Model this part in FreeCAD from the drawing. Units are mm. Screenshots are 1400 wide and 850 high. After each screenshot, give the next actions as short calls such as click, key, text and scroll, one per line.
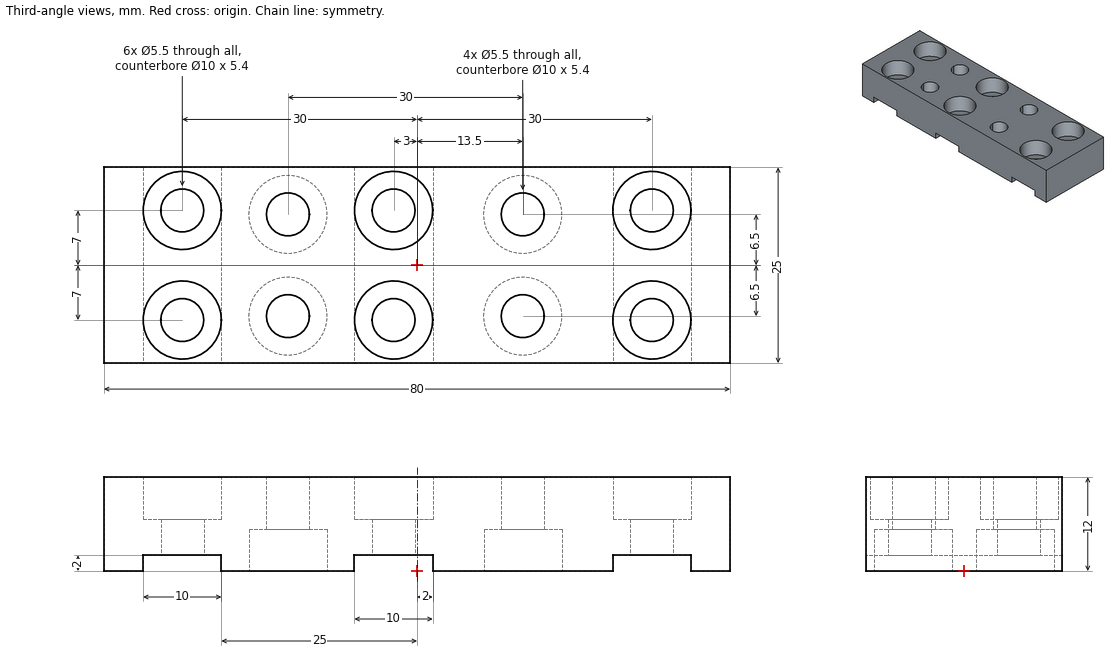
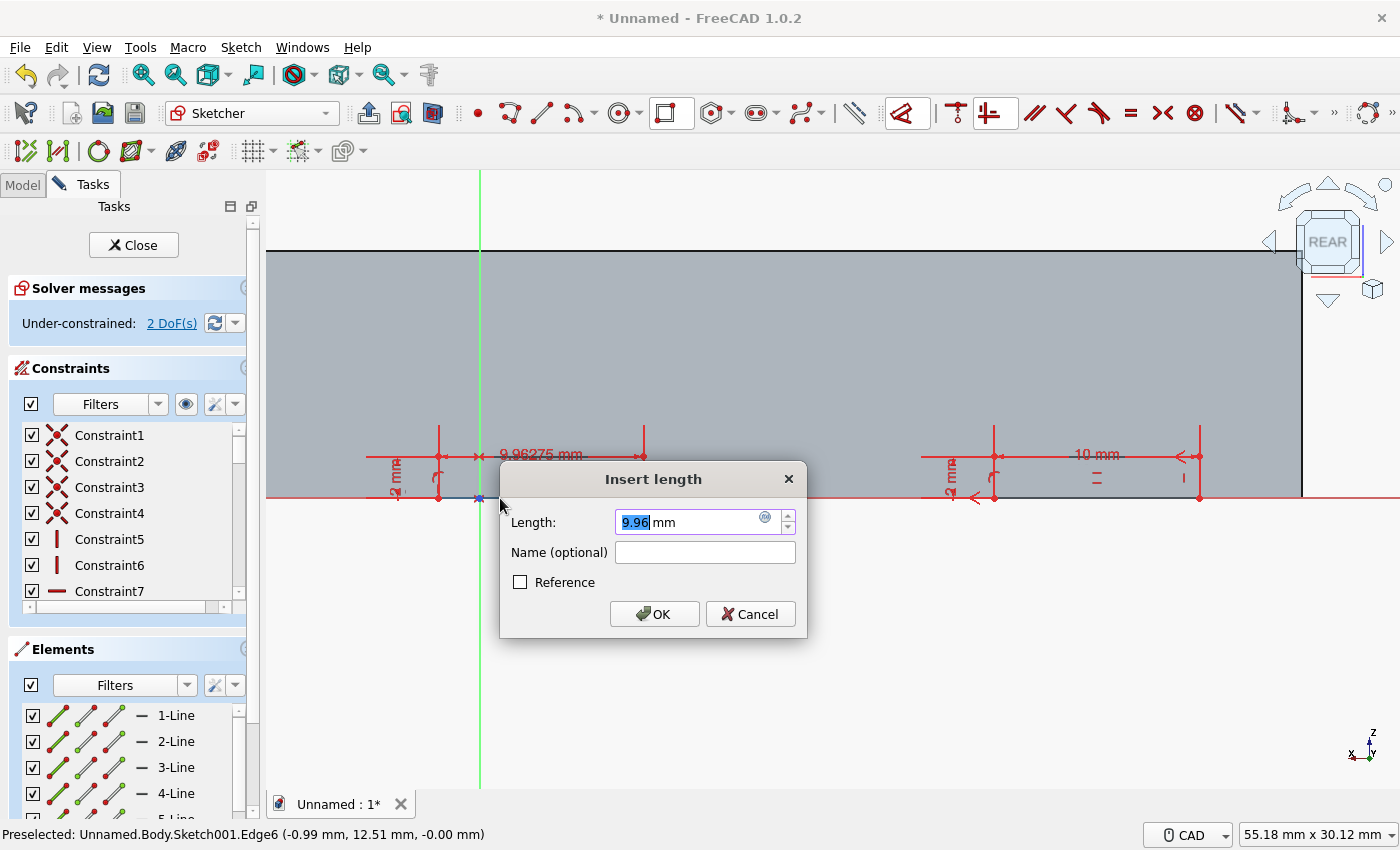
text(10)
key(Return)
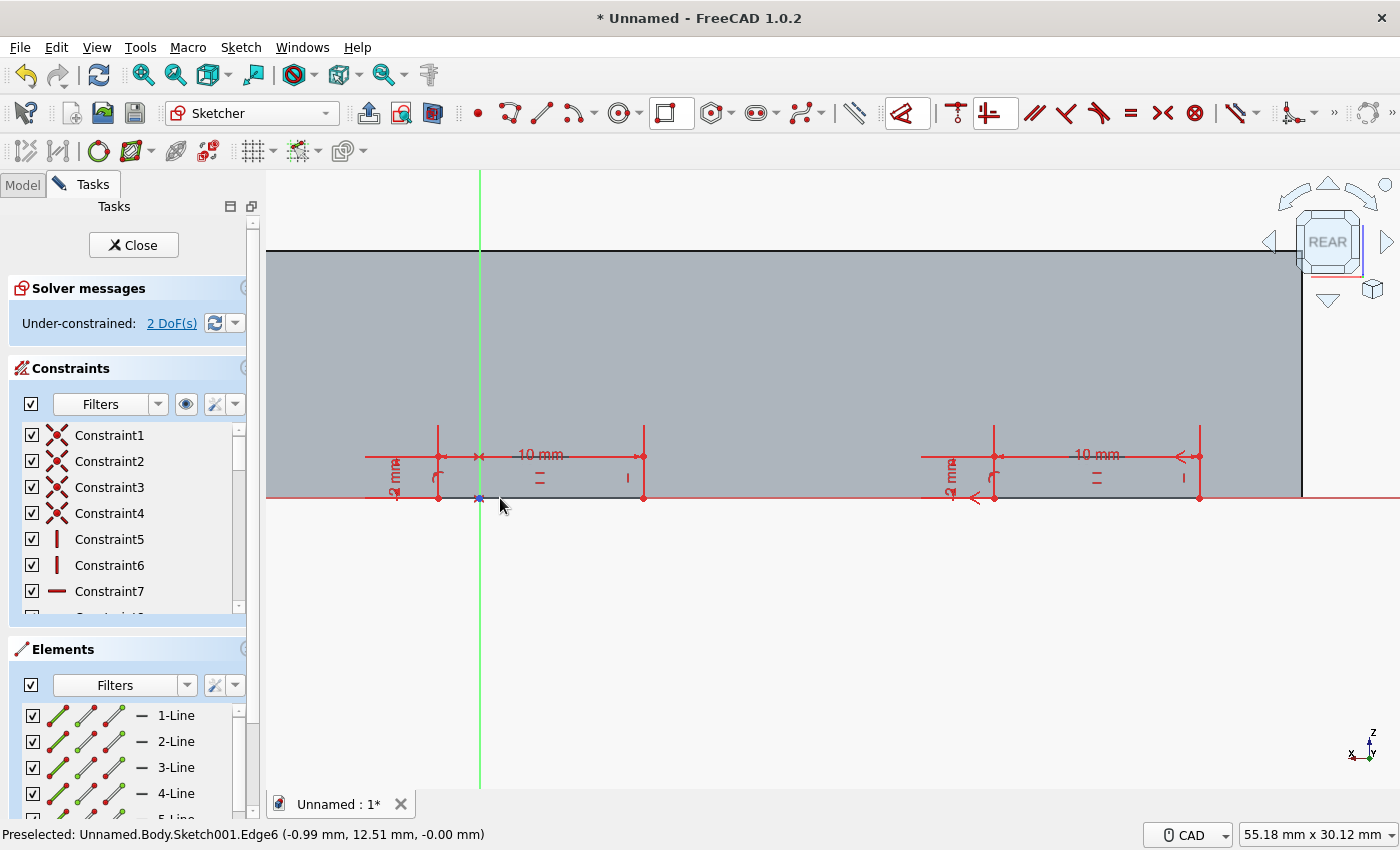
click(438, 457)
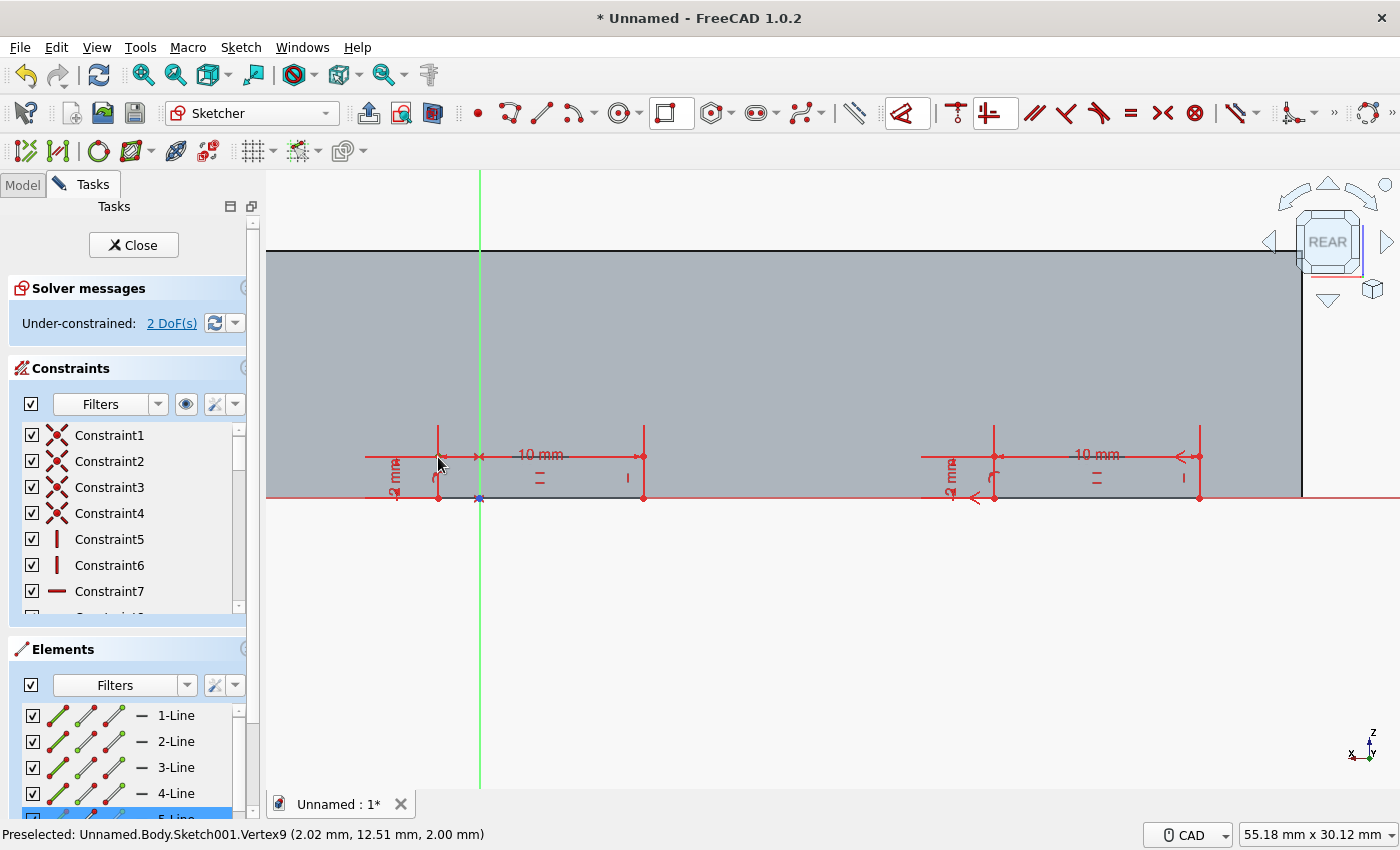
click(924, 114)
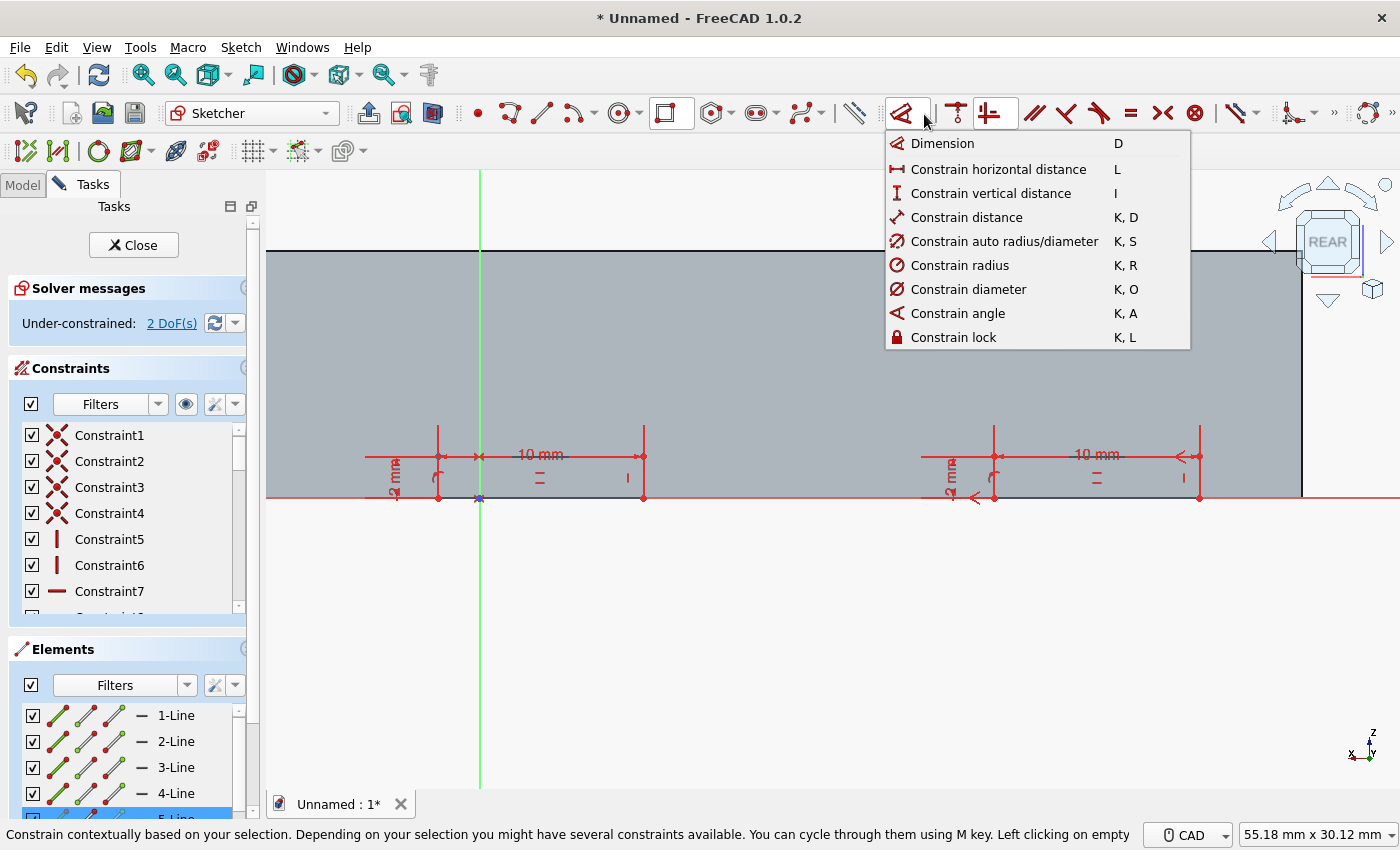
click(1038, 169)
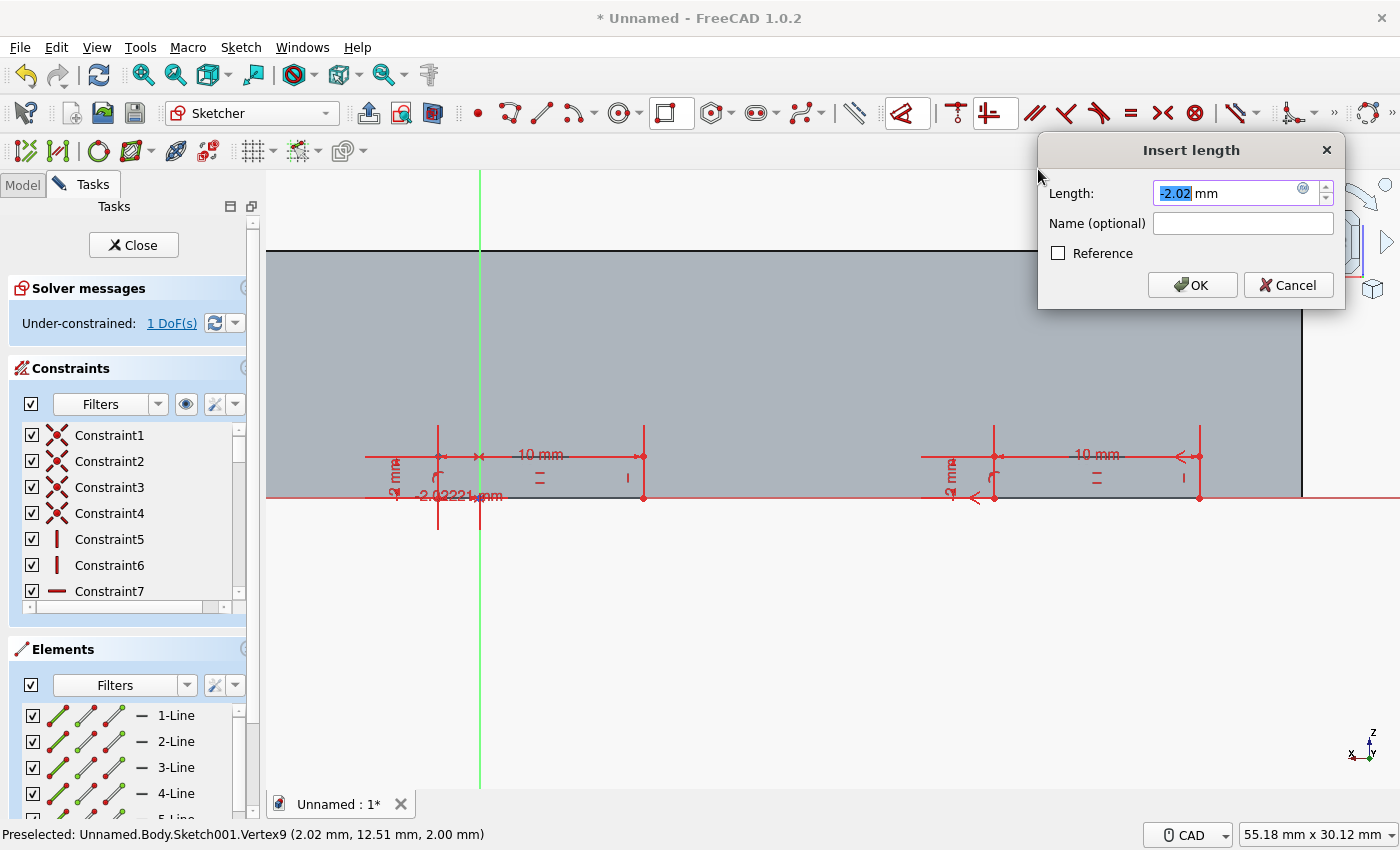
text(-2)
key(Return)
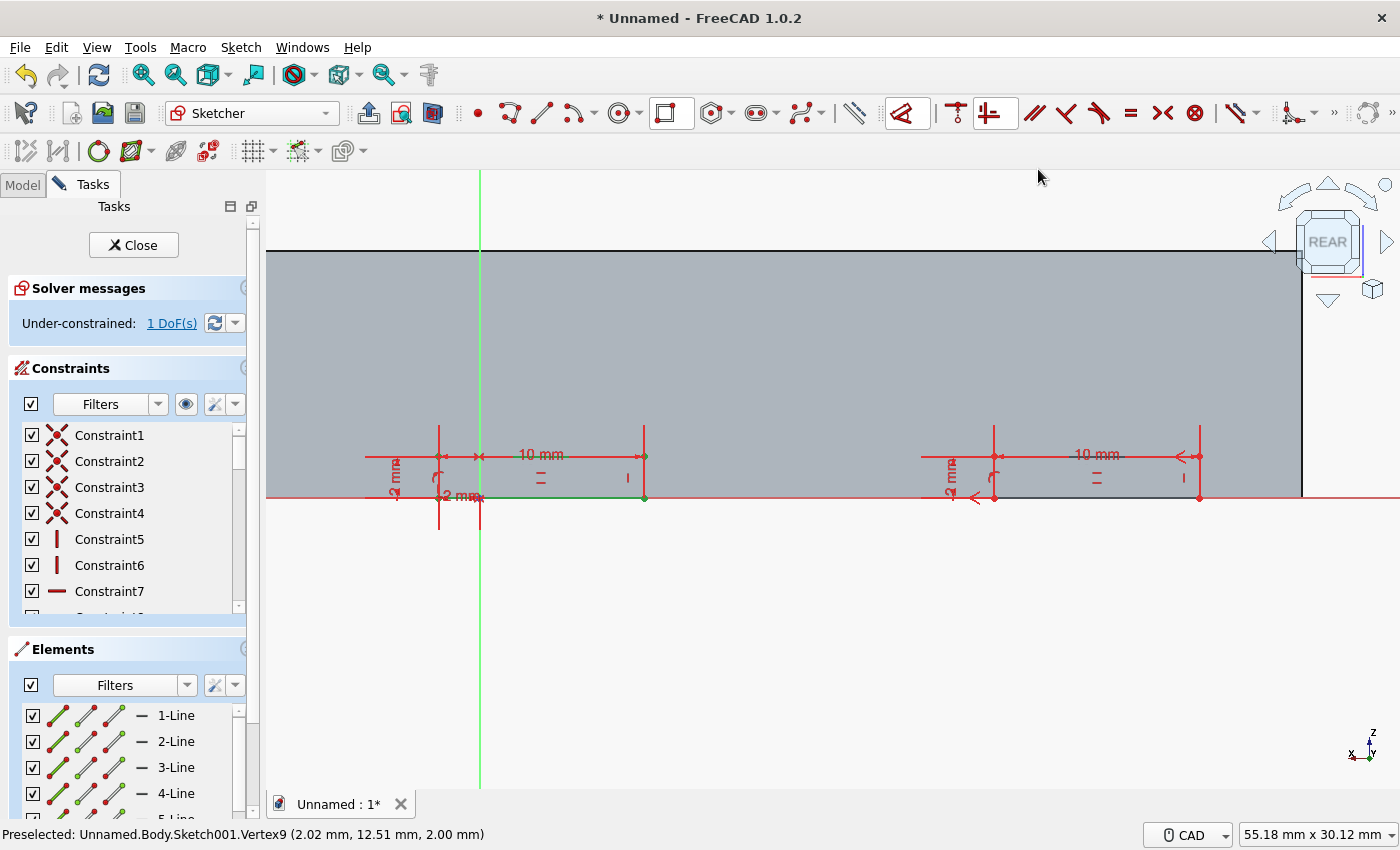
click(994, 457)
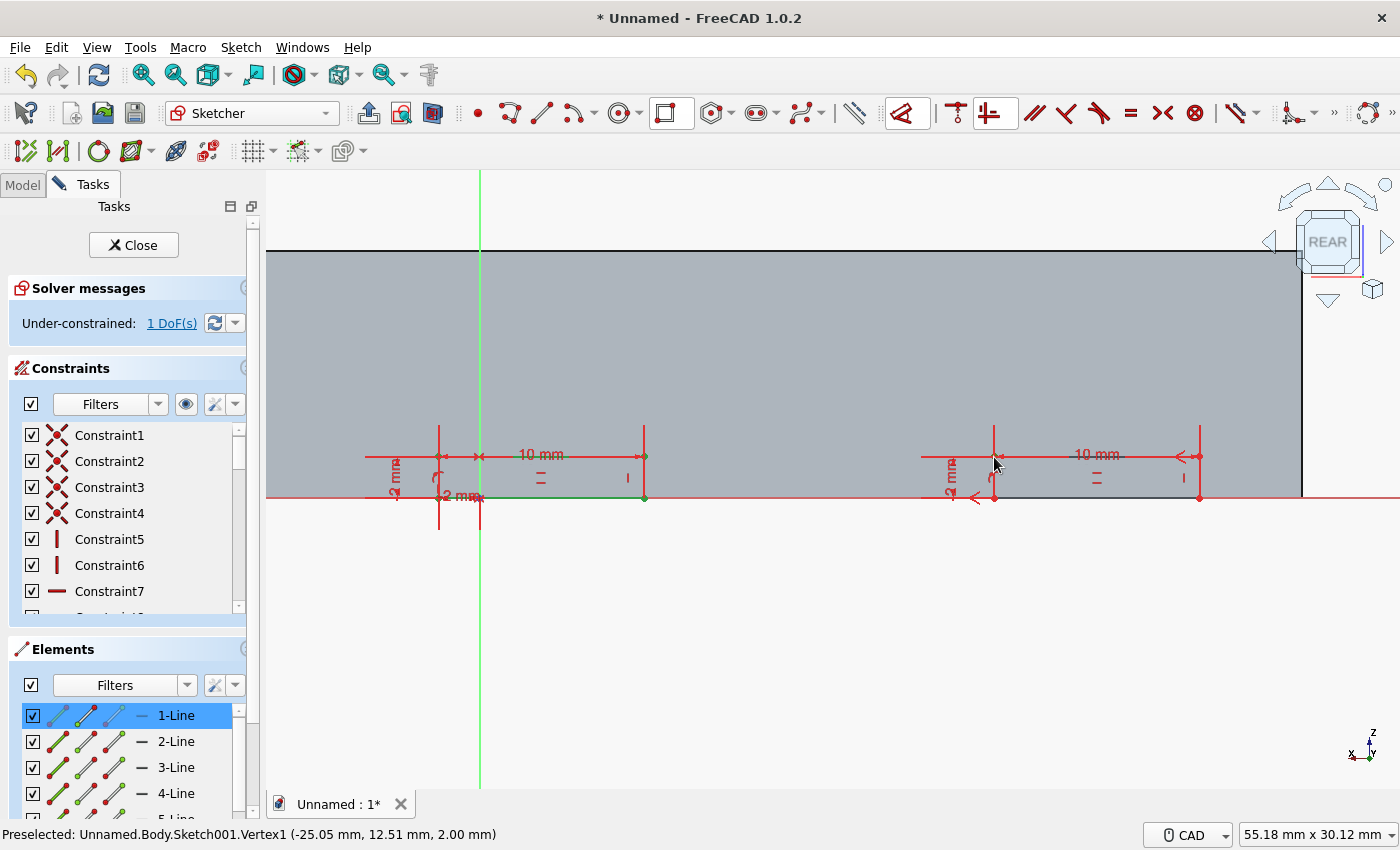
key(l)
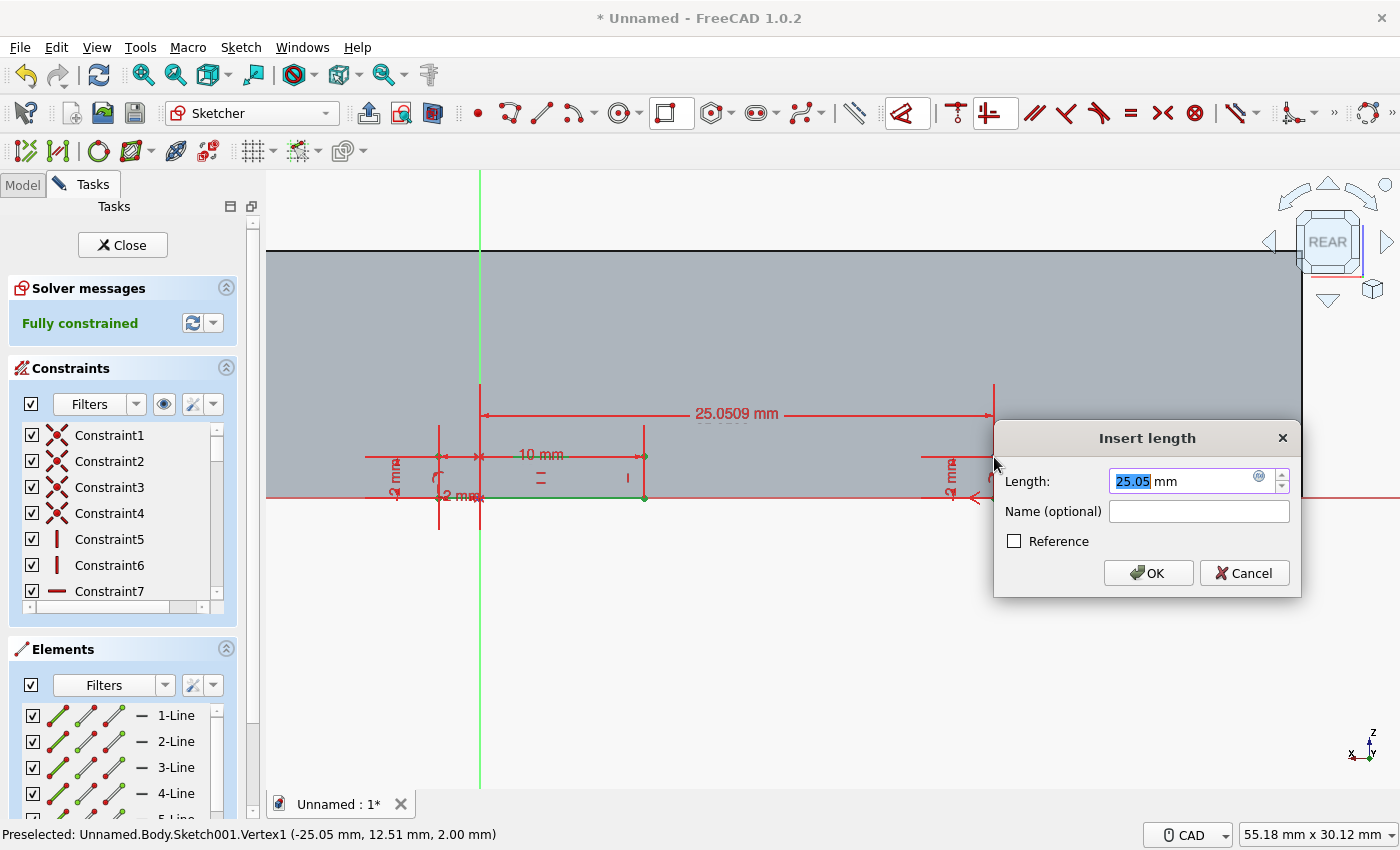
text(25)
key(Return)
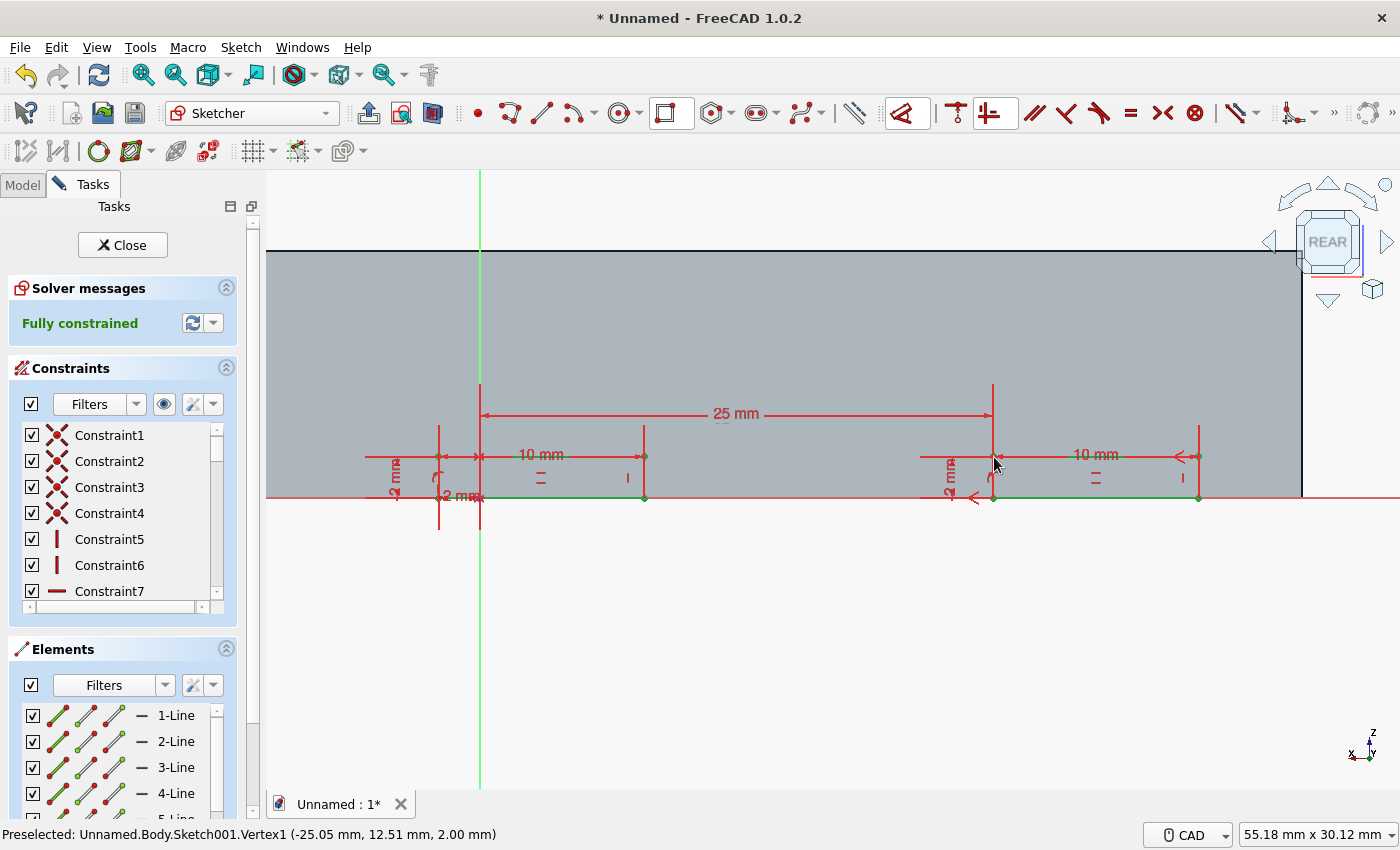
click(123, 245)